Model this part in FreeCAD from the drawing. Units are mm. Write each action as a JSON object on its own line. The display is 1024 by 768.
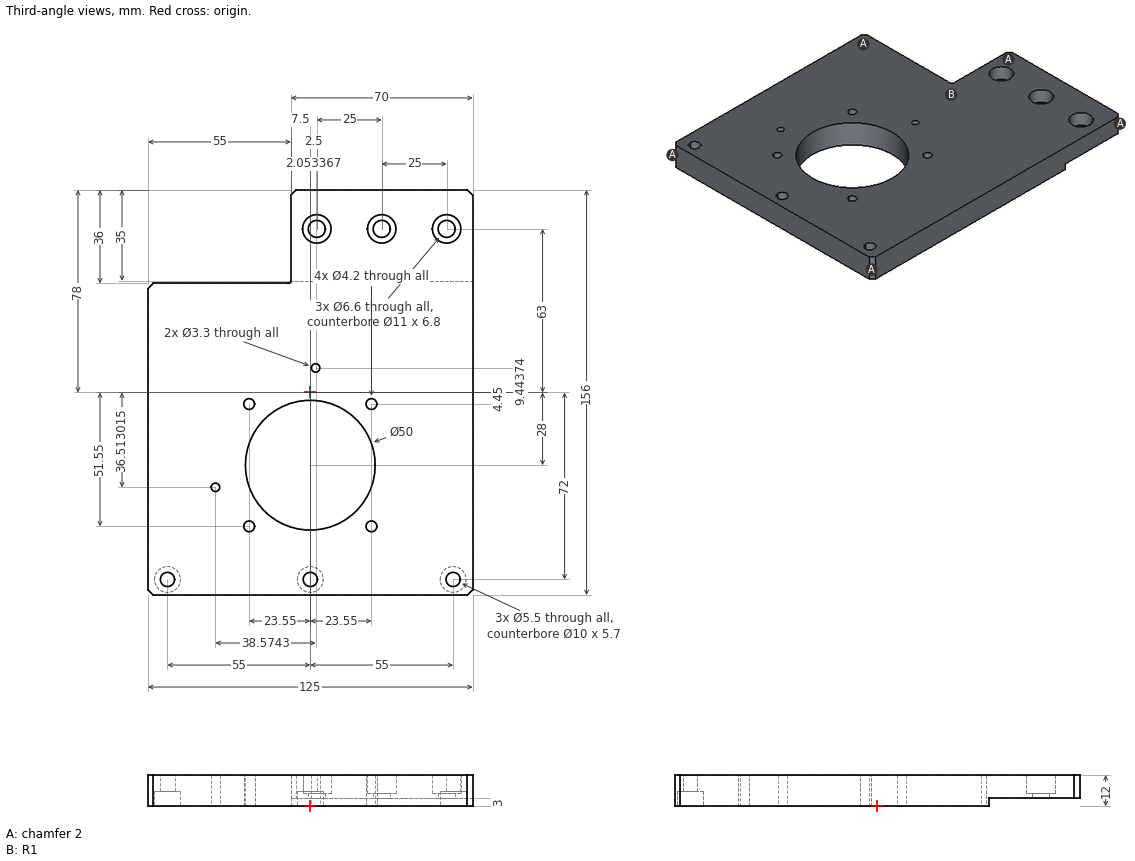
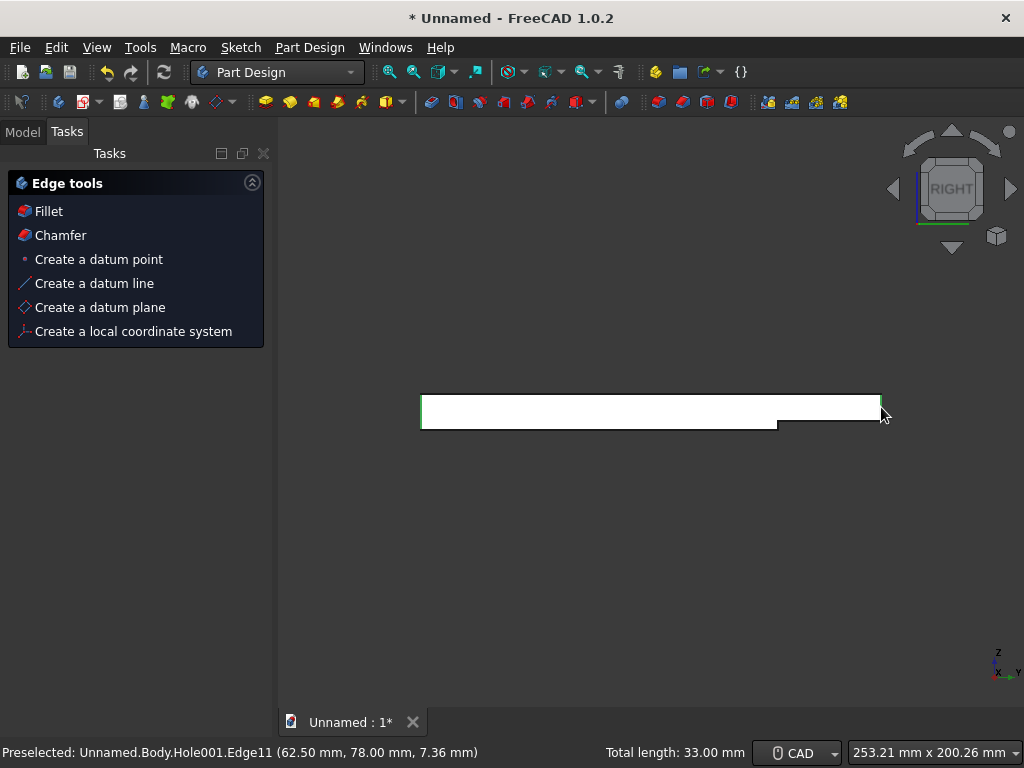
{"action": "key", "text": "5"}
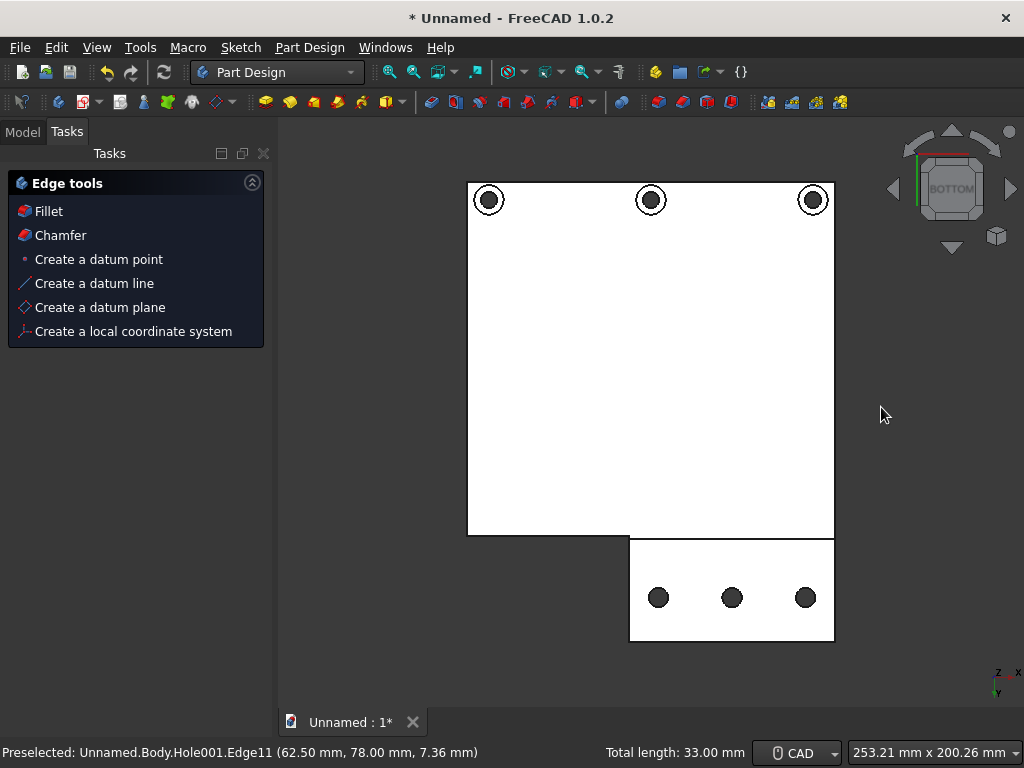
{"action": "key", "text": "4"}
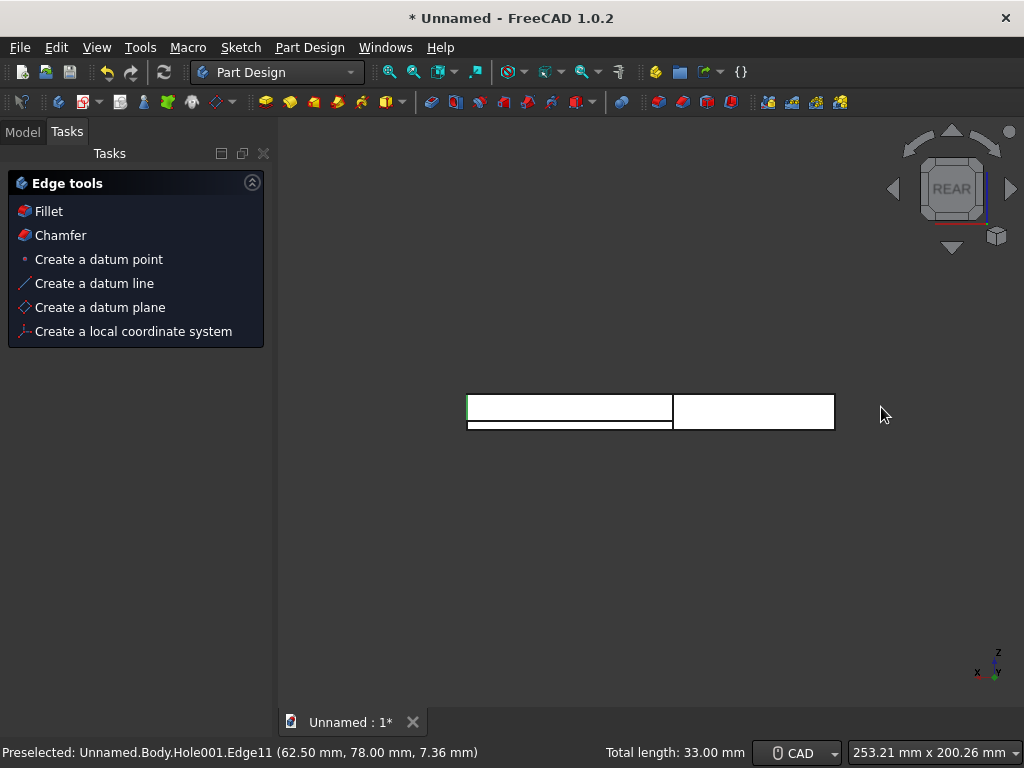
{"action": "left_click", "coordinate": [835, 411], "text": "ctrl"}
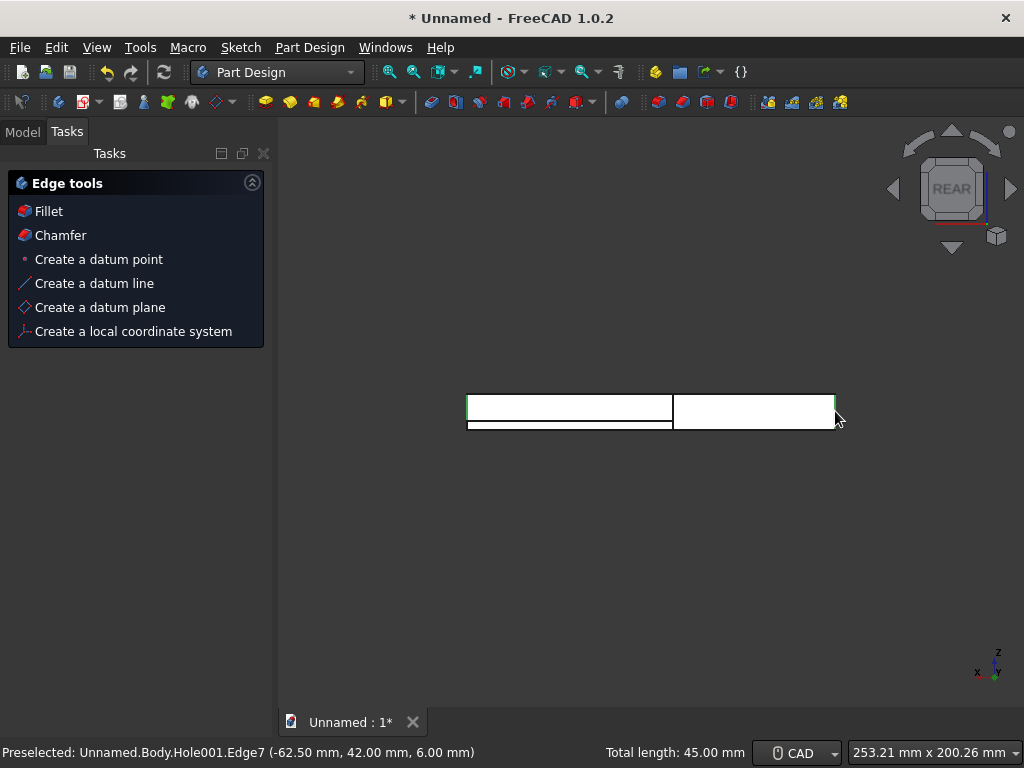
{"action": "left_click", "coordinate": [673, 407], "text": "ctrl"}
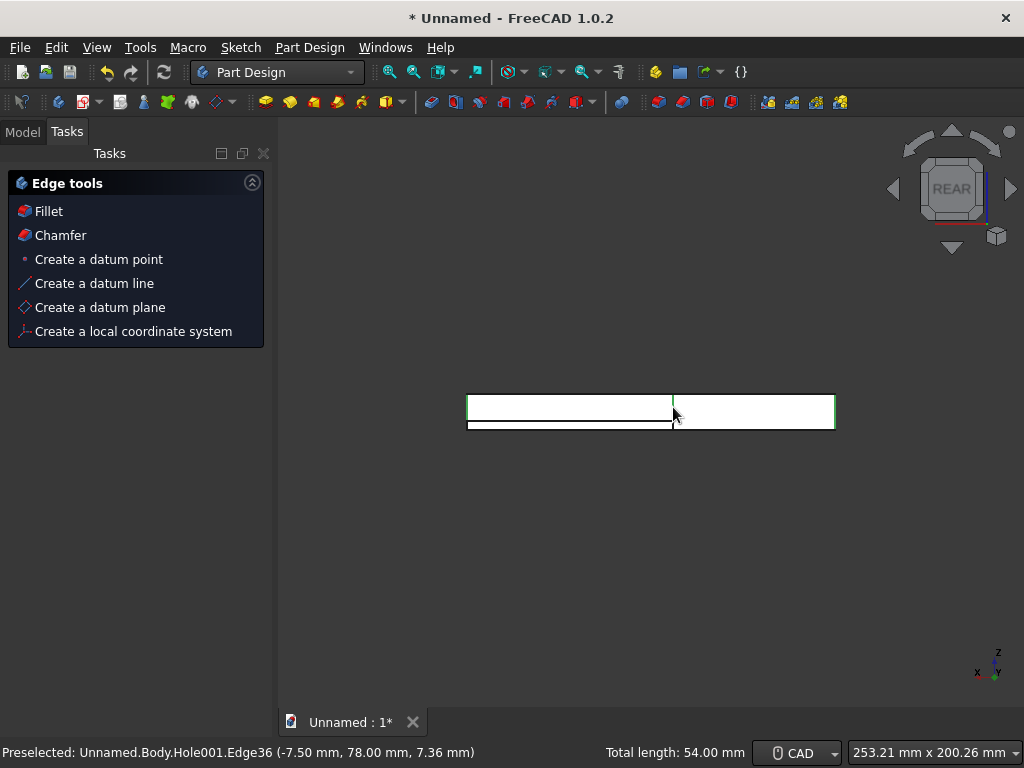
{"action": "left_click", "coordinate": [684, 102]}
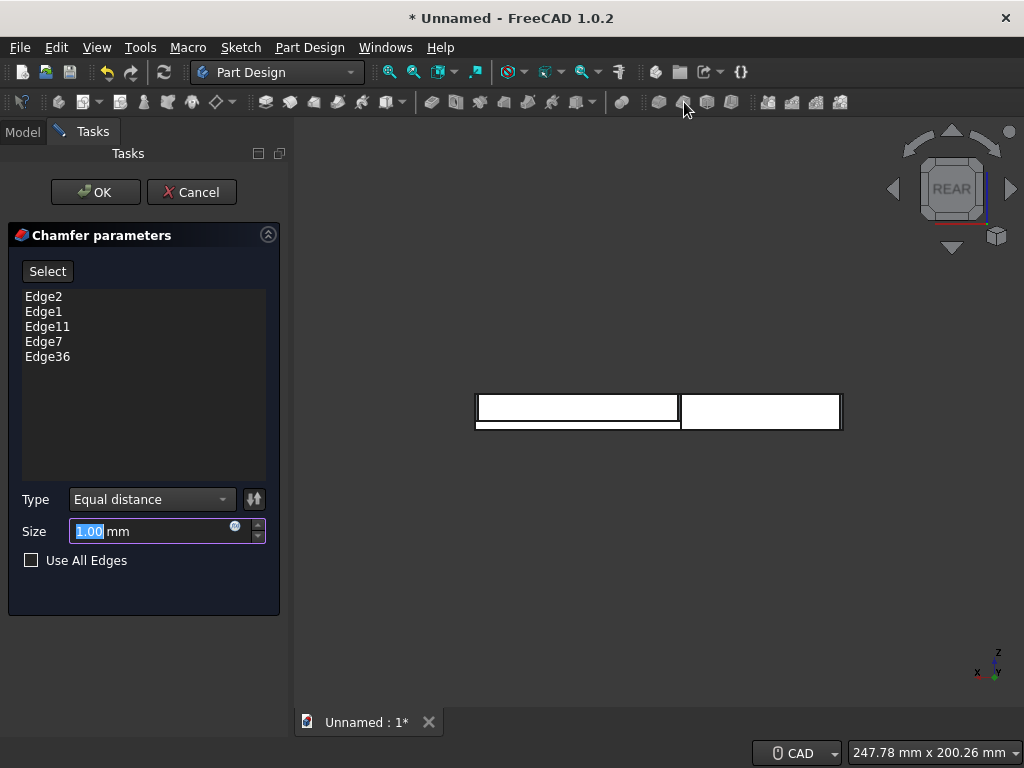
{"action": "type", "text": "2"}
{"action": "key", "text": "Tab"}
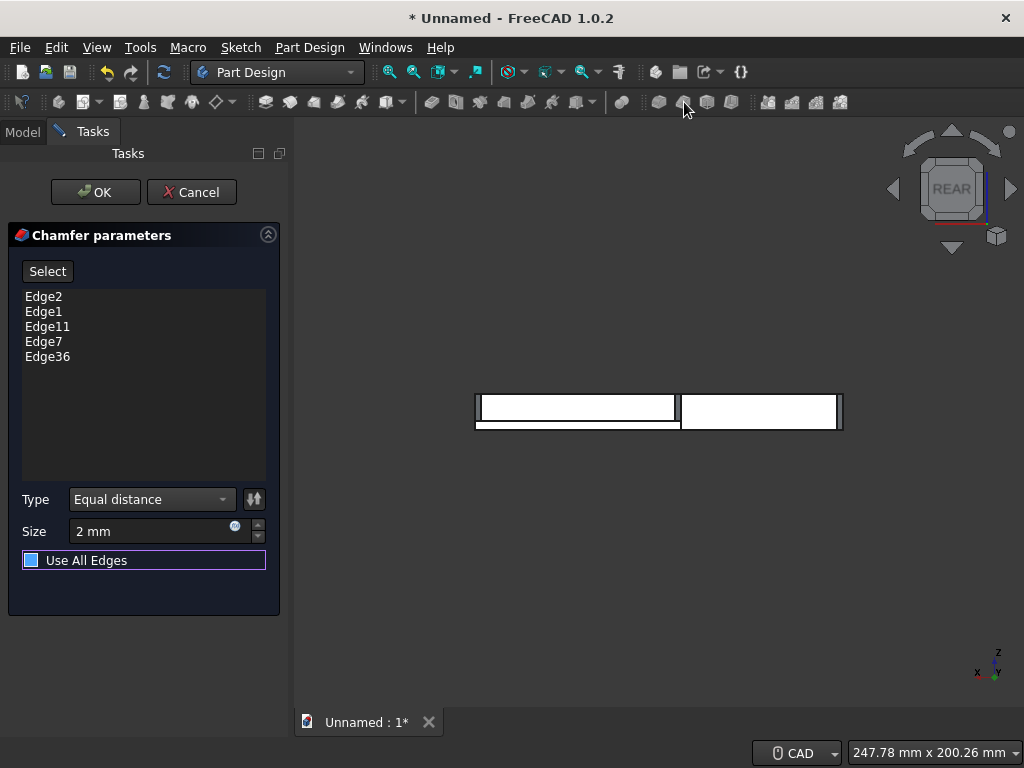
{"action": "left_click", "coordinate": [96, 192]}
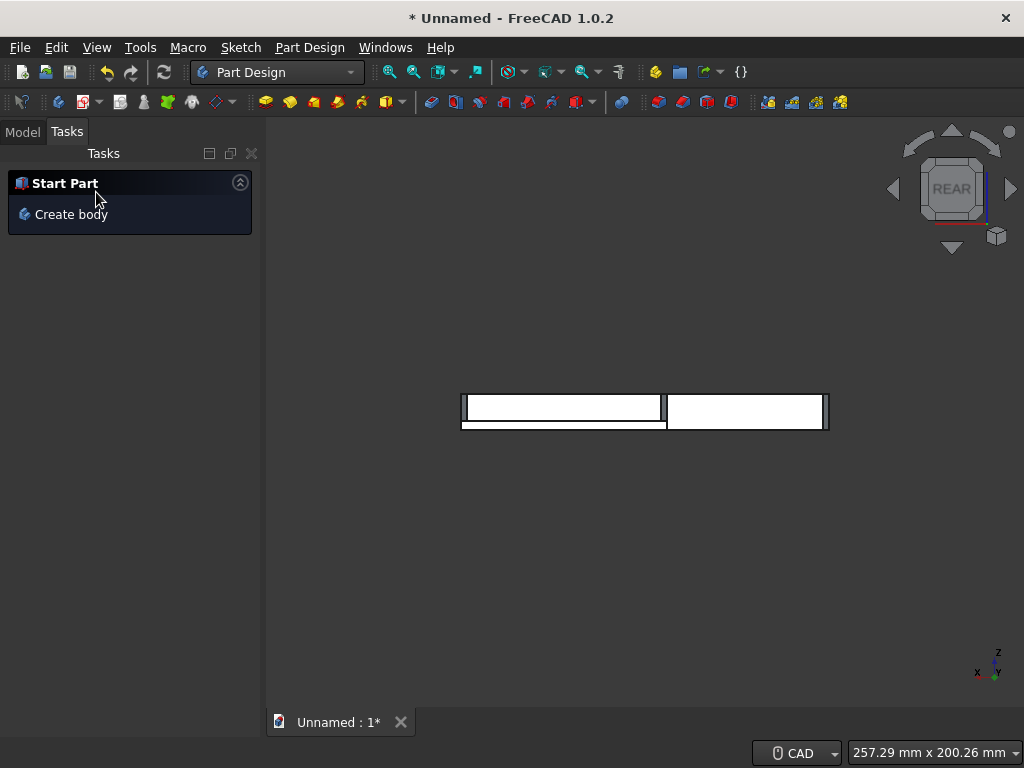
{"action": "key", "text": "0"}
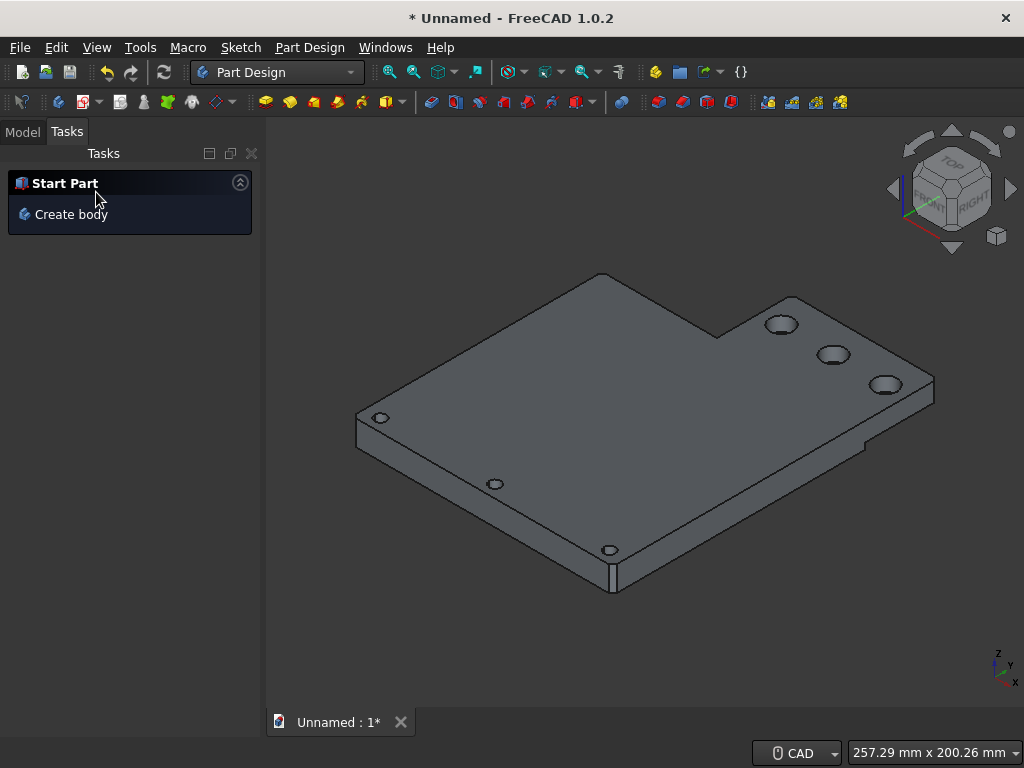
{"action": "key", "text": "2"}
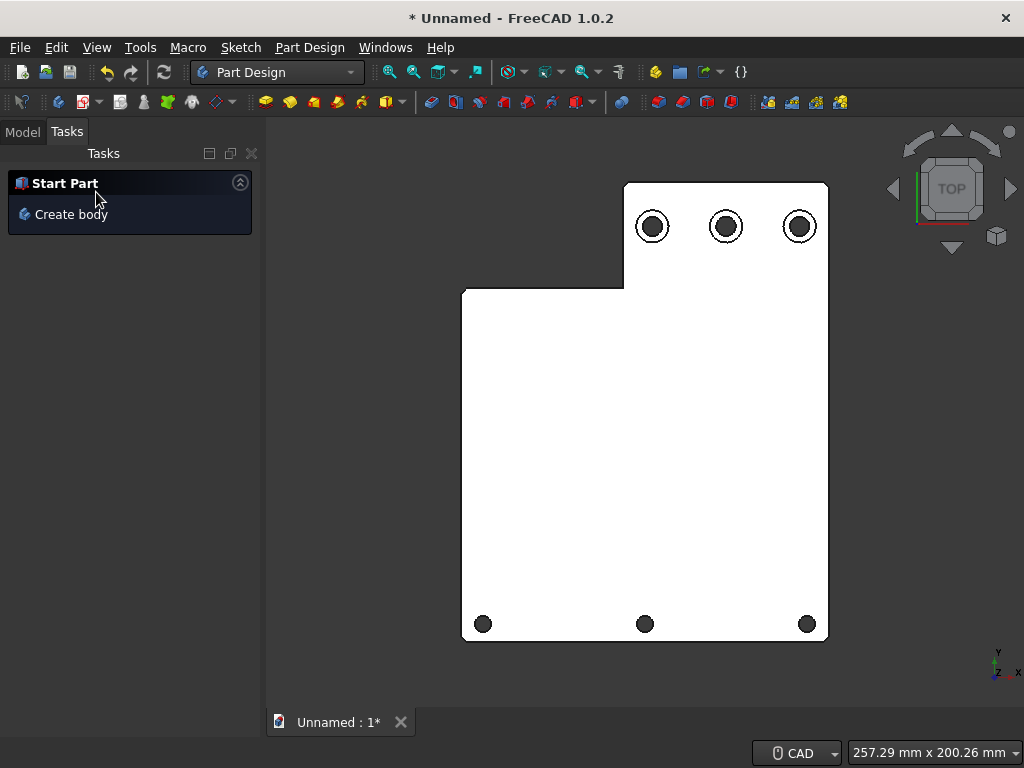
{"action": "key", "text": "1"}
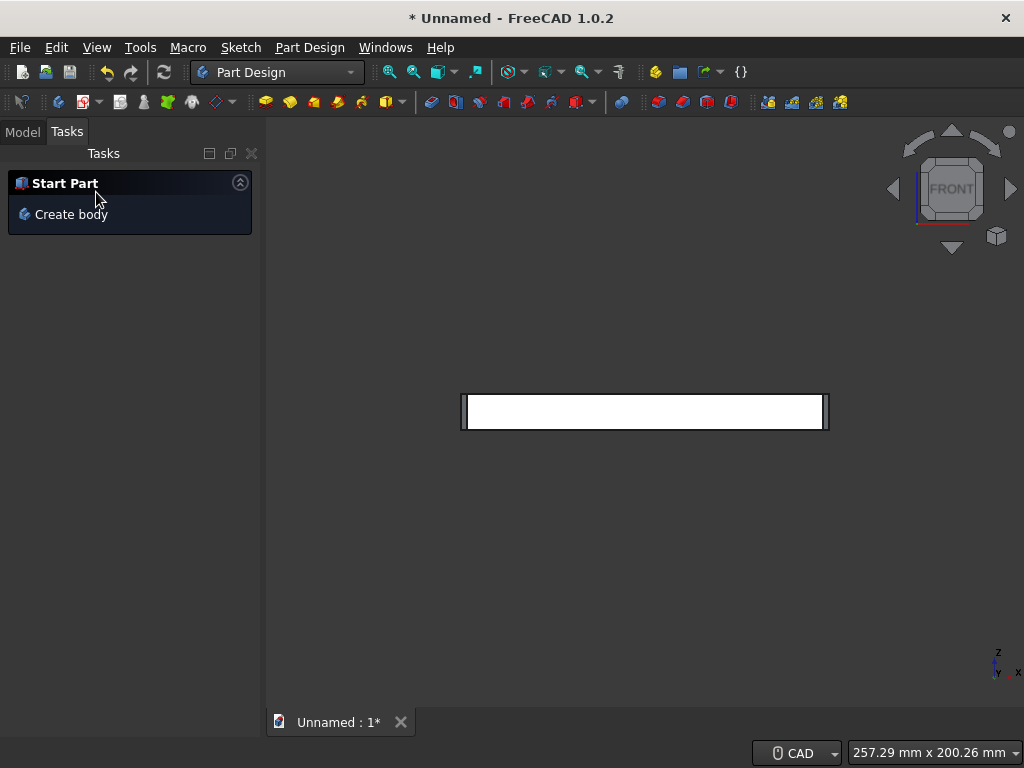
{"action": "key", "text": "3"}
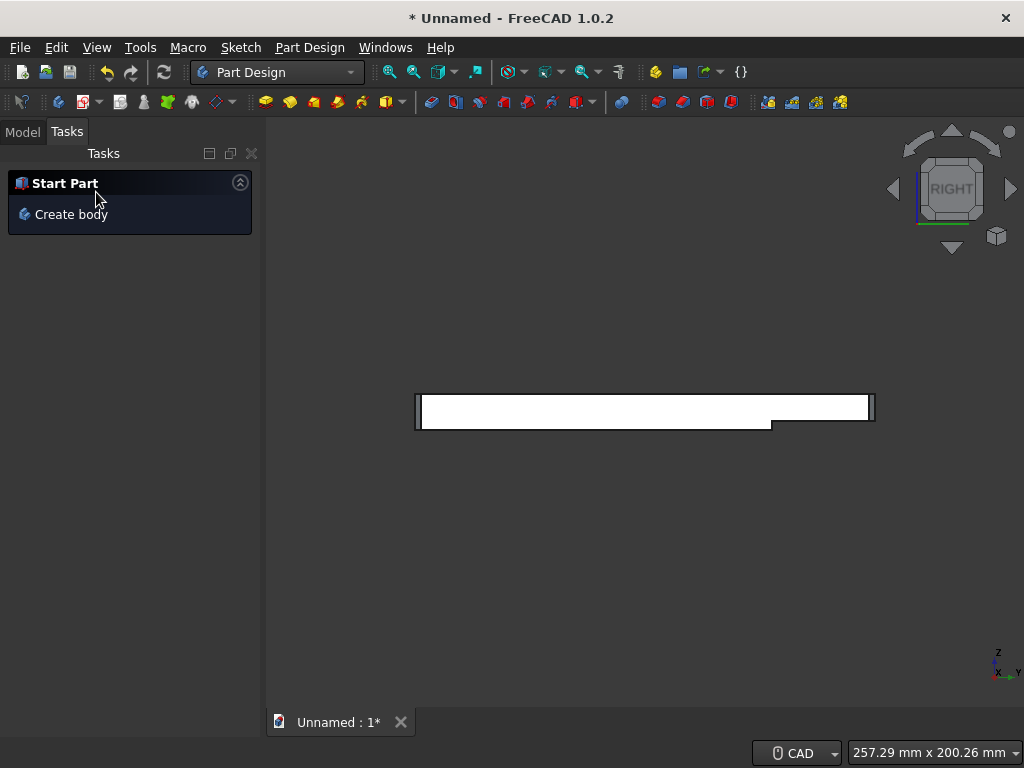
{"action": "key", "text": "5"}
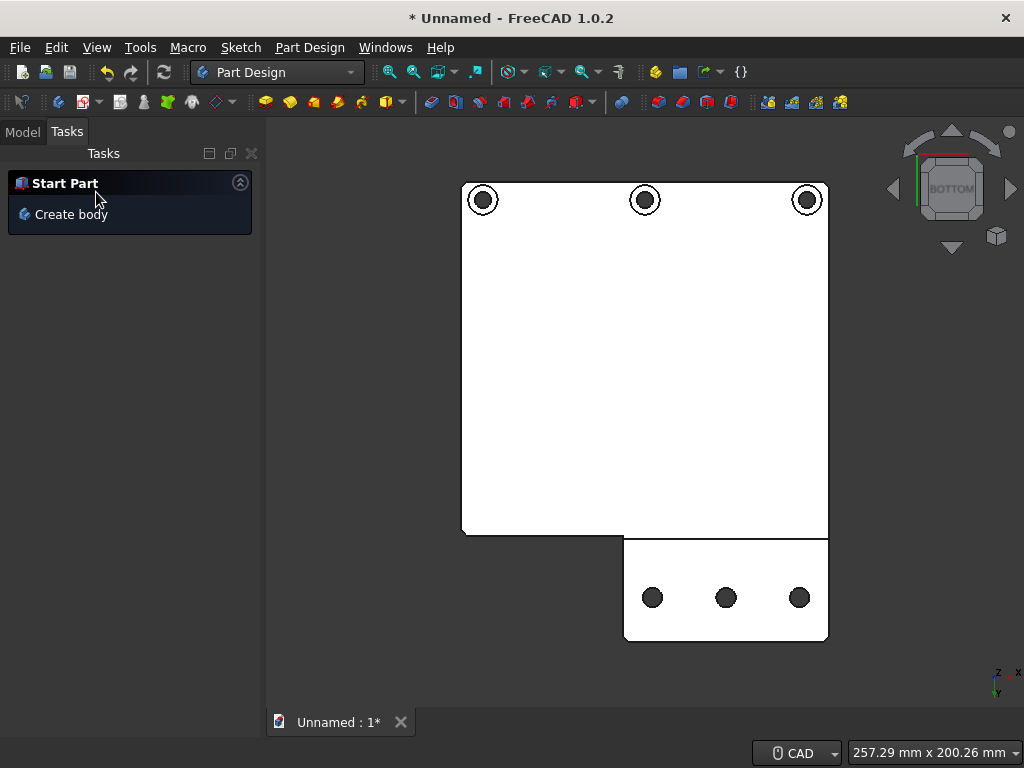
{"action": "key", "text": "4"}